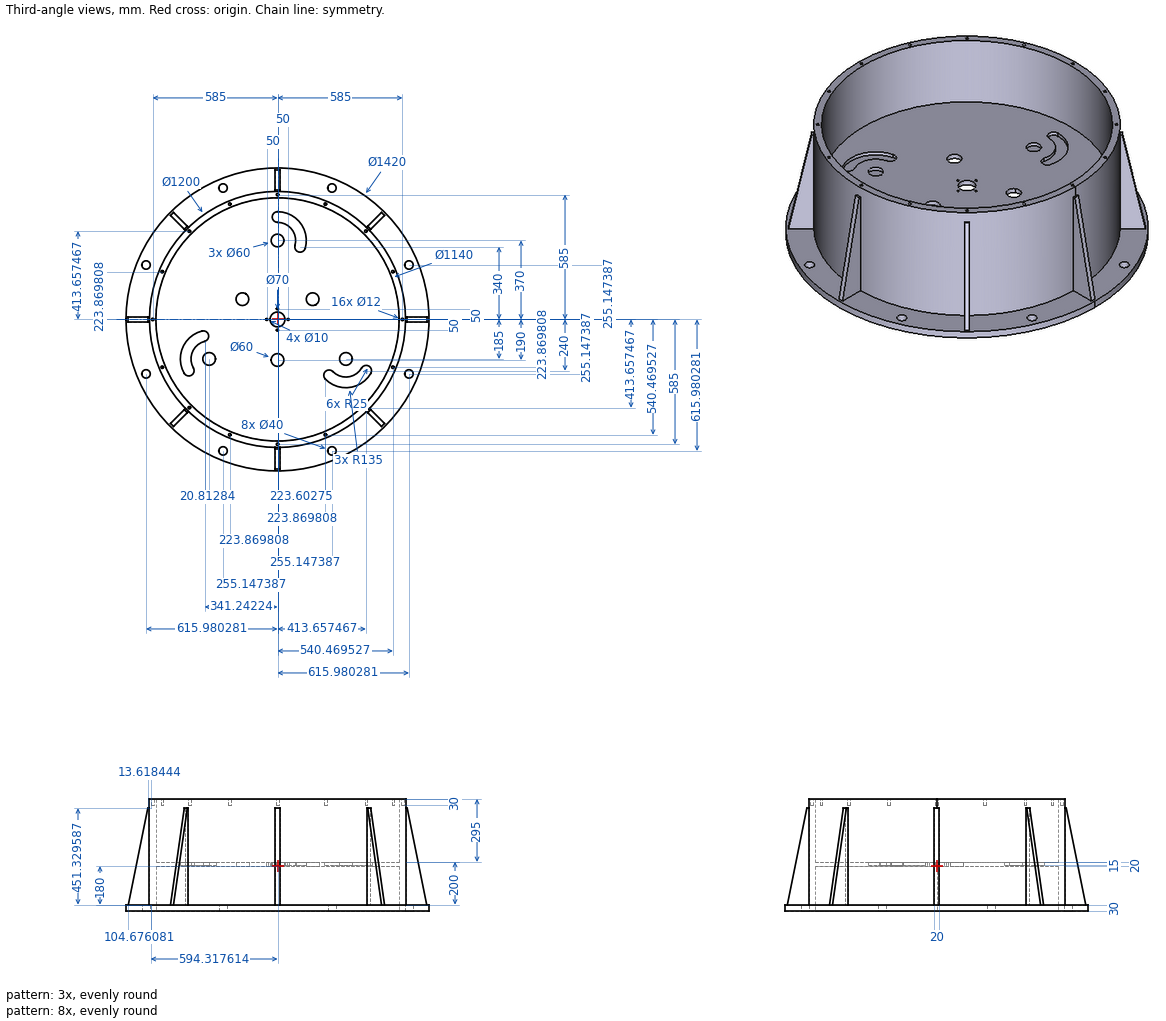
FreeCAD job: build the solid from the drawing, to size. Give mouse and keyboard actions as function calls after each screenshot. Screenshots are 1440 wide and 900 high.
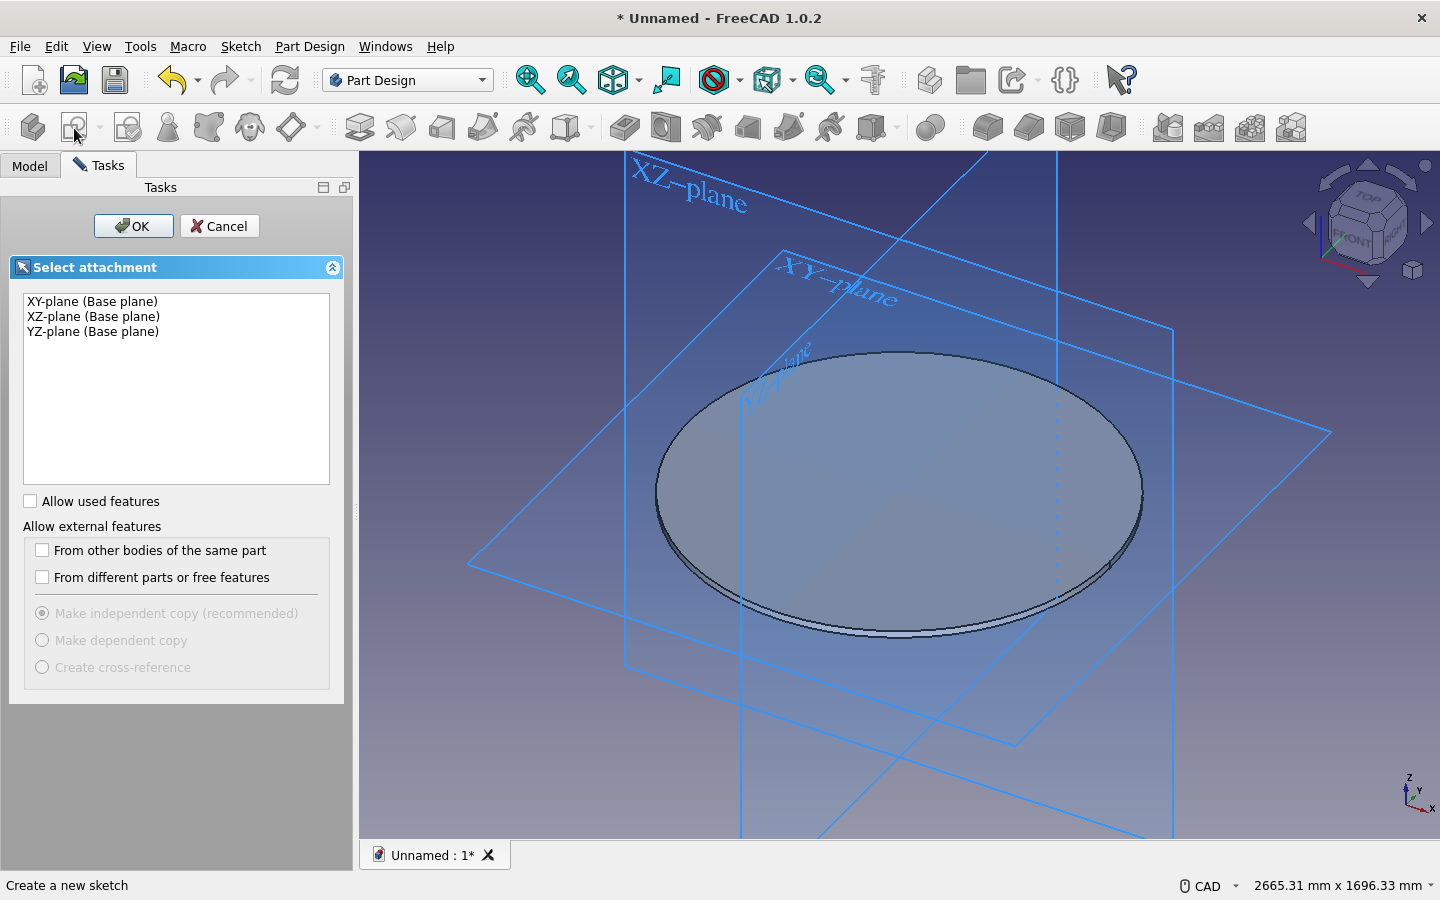
click(84, 302)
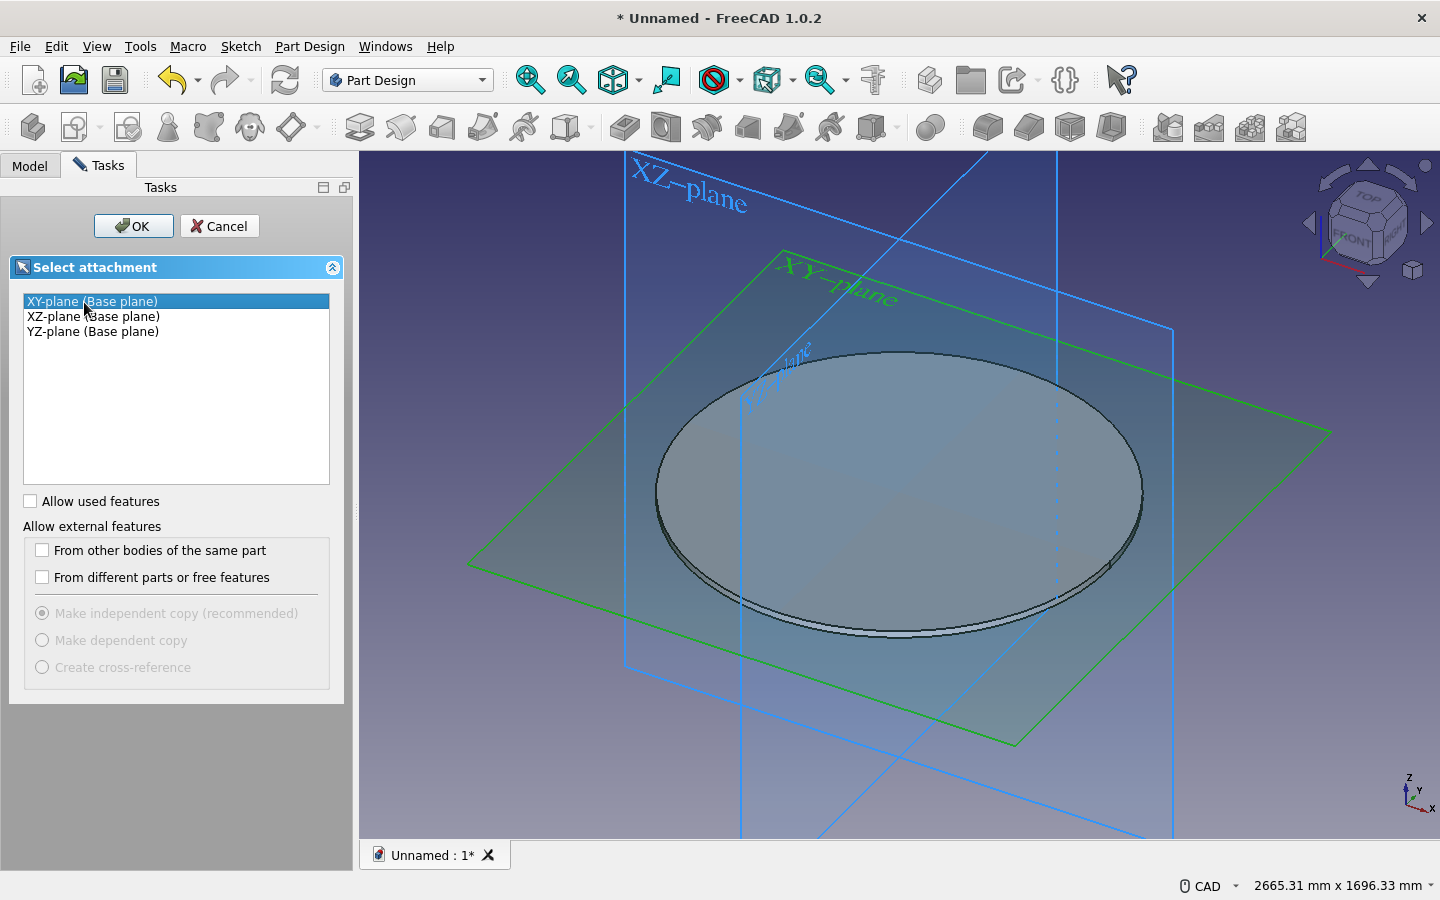
click(134, 226)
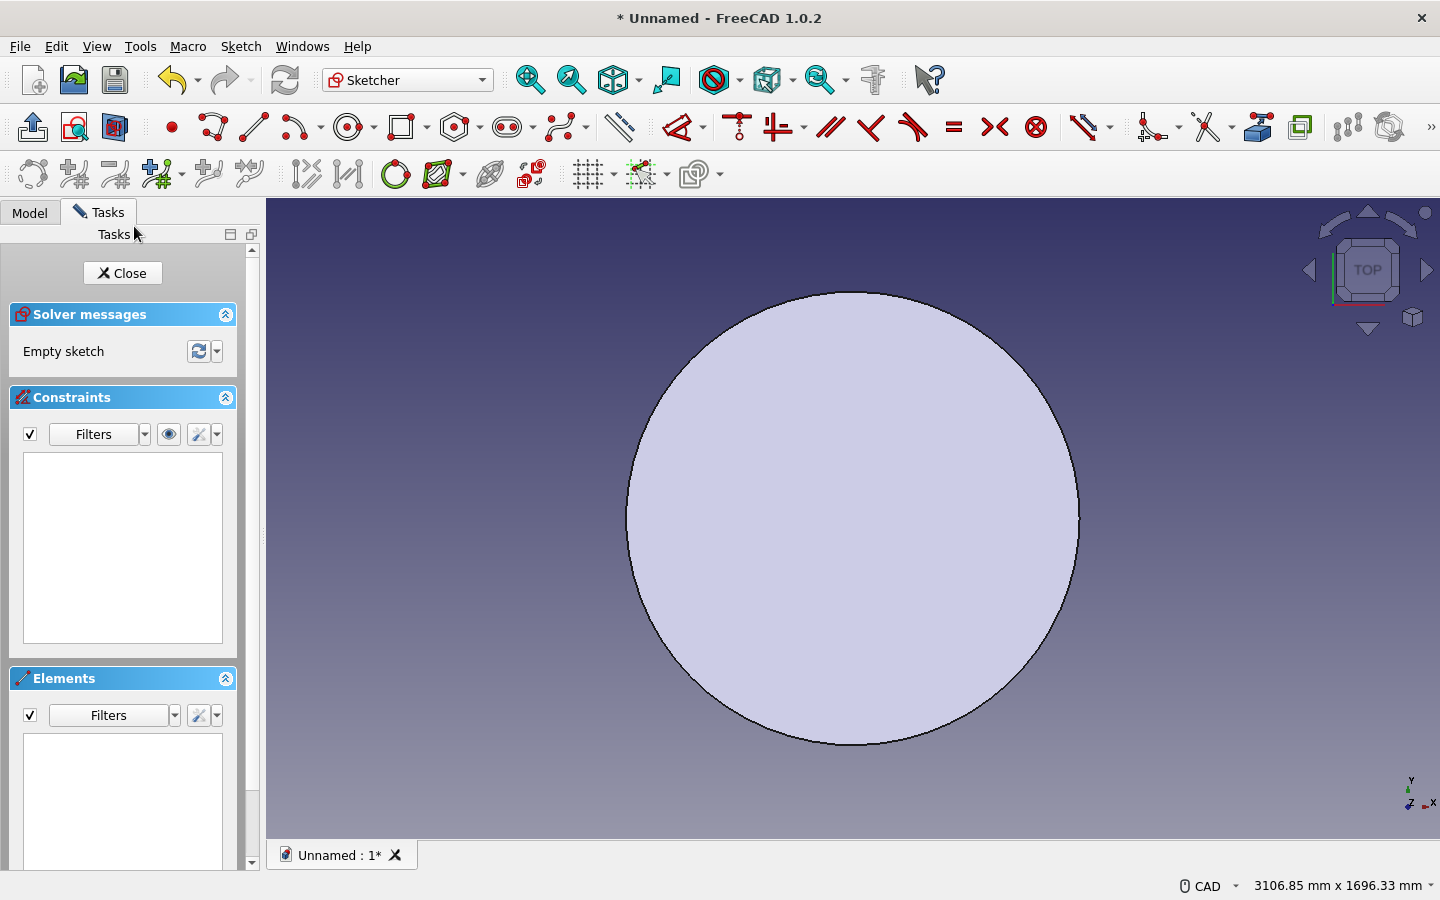
key(q)
key(s)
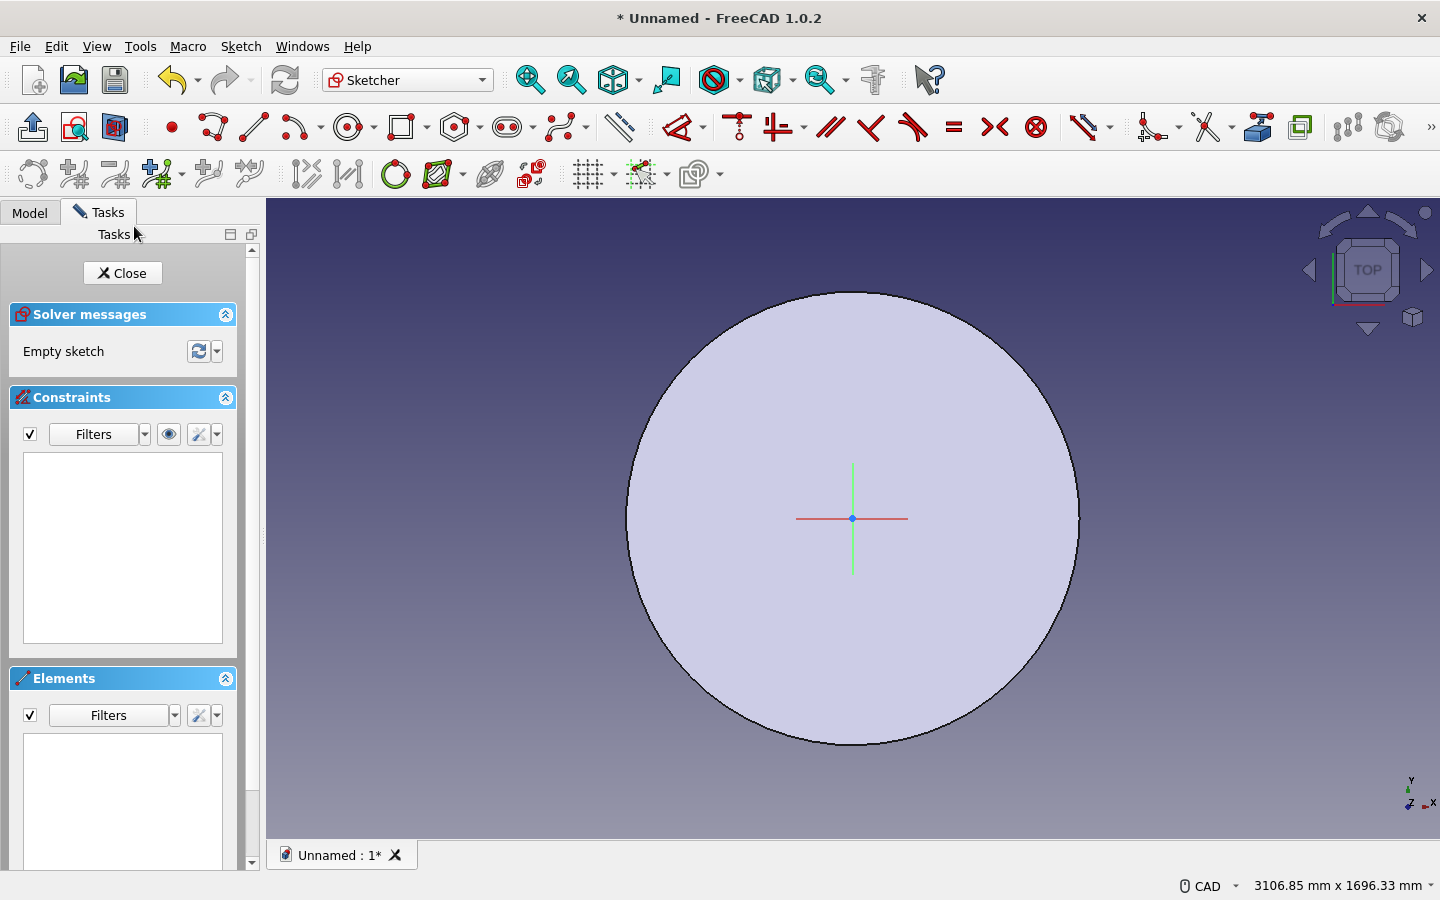
scroll(861, 518, up, 11)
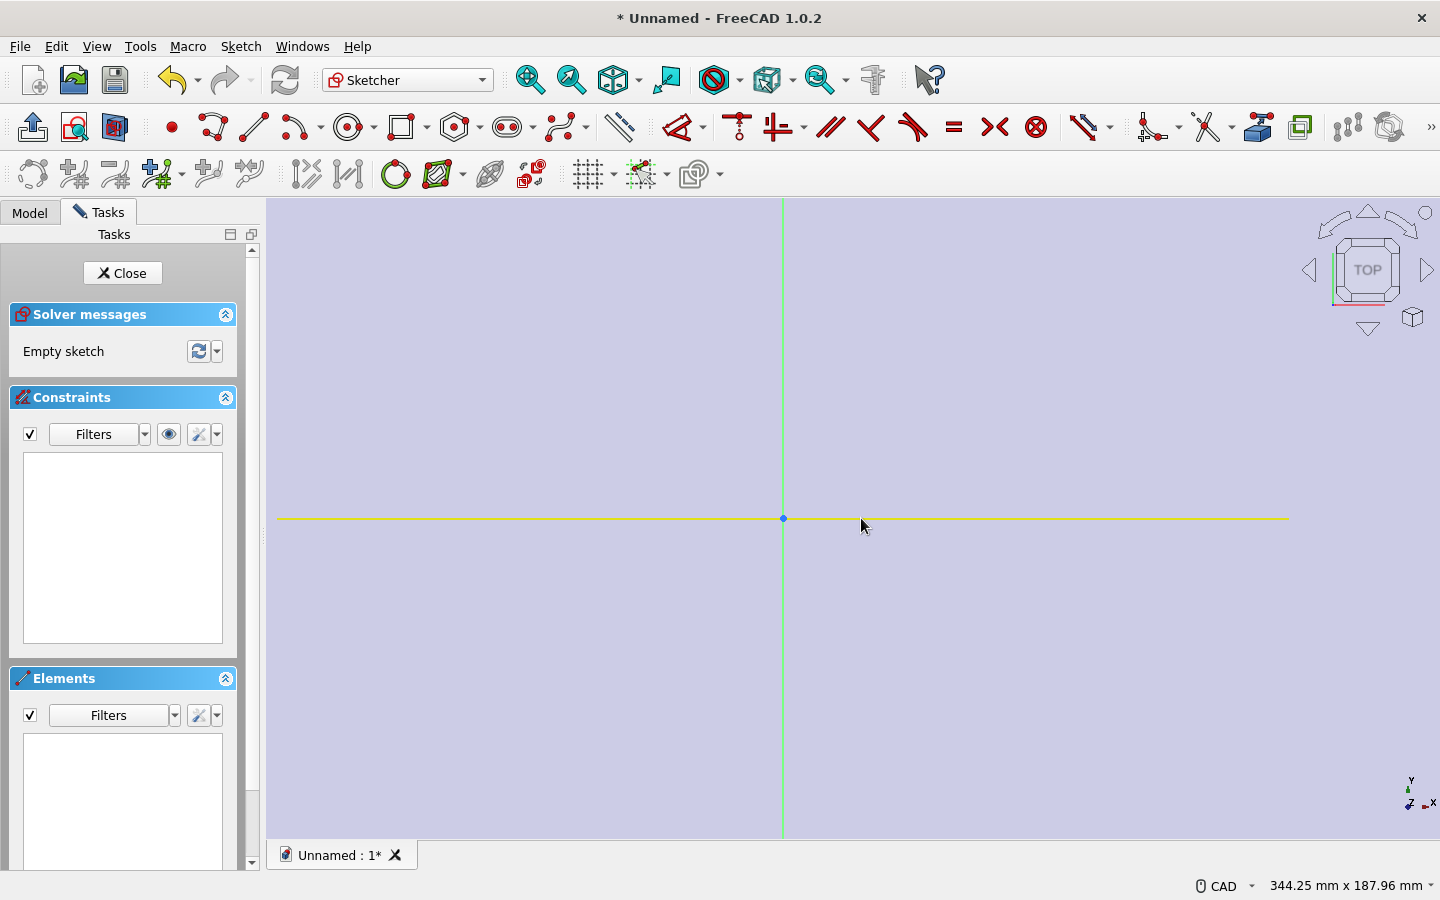
key(g)
key(c)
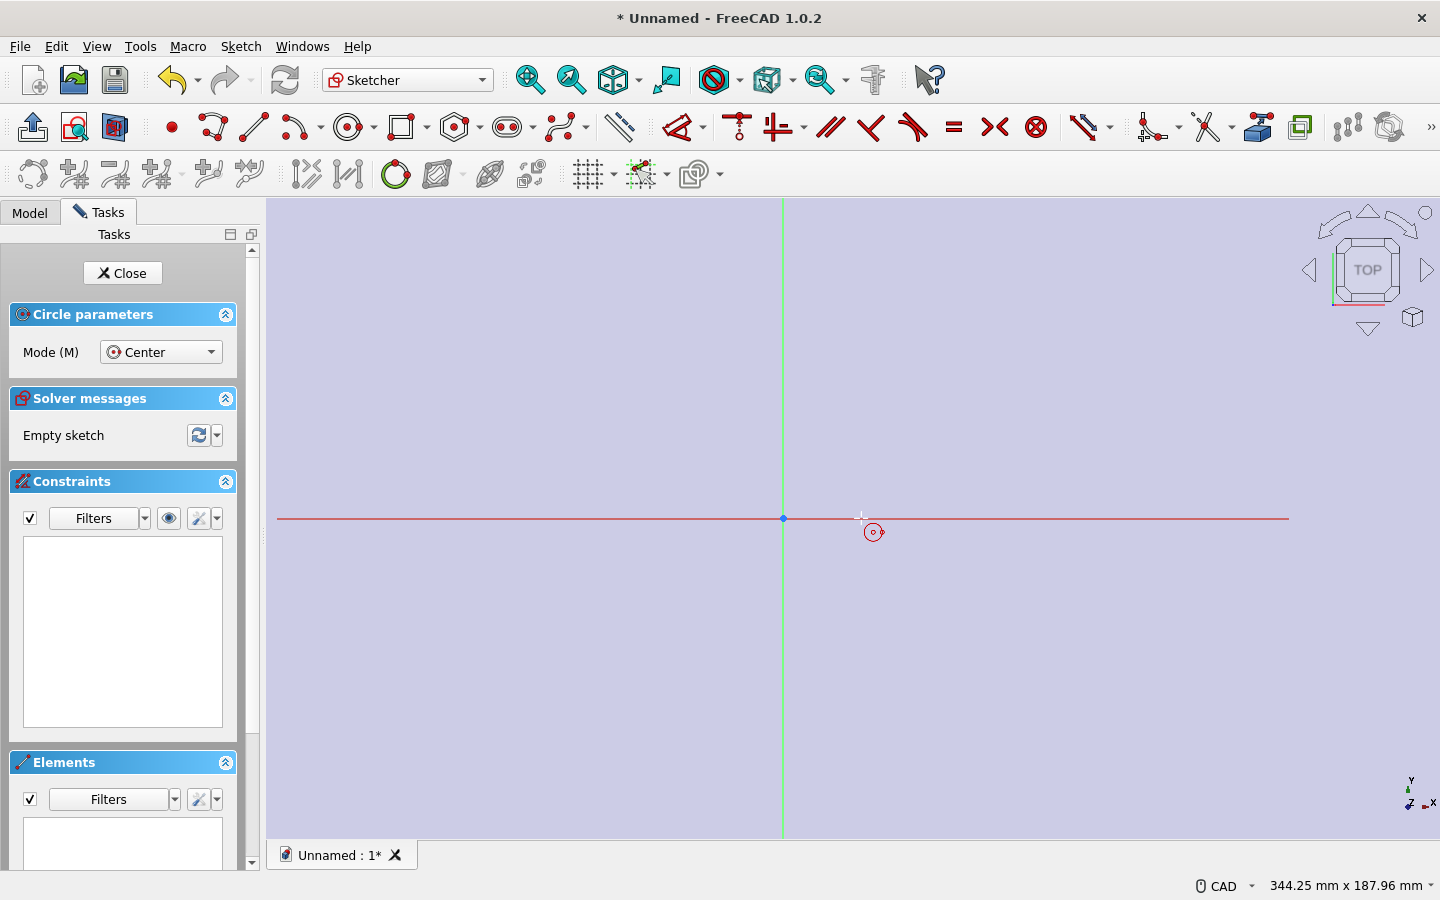
click(783, 518)
move(868, 434)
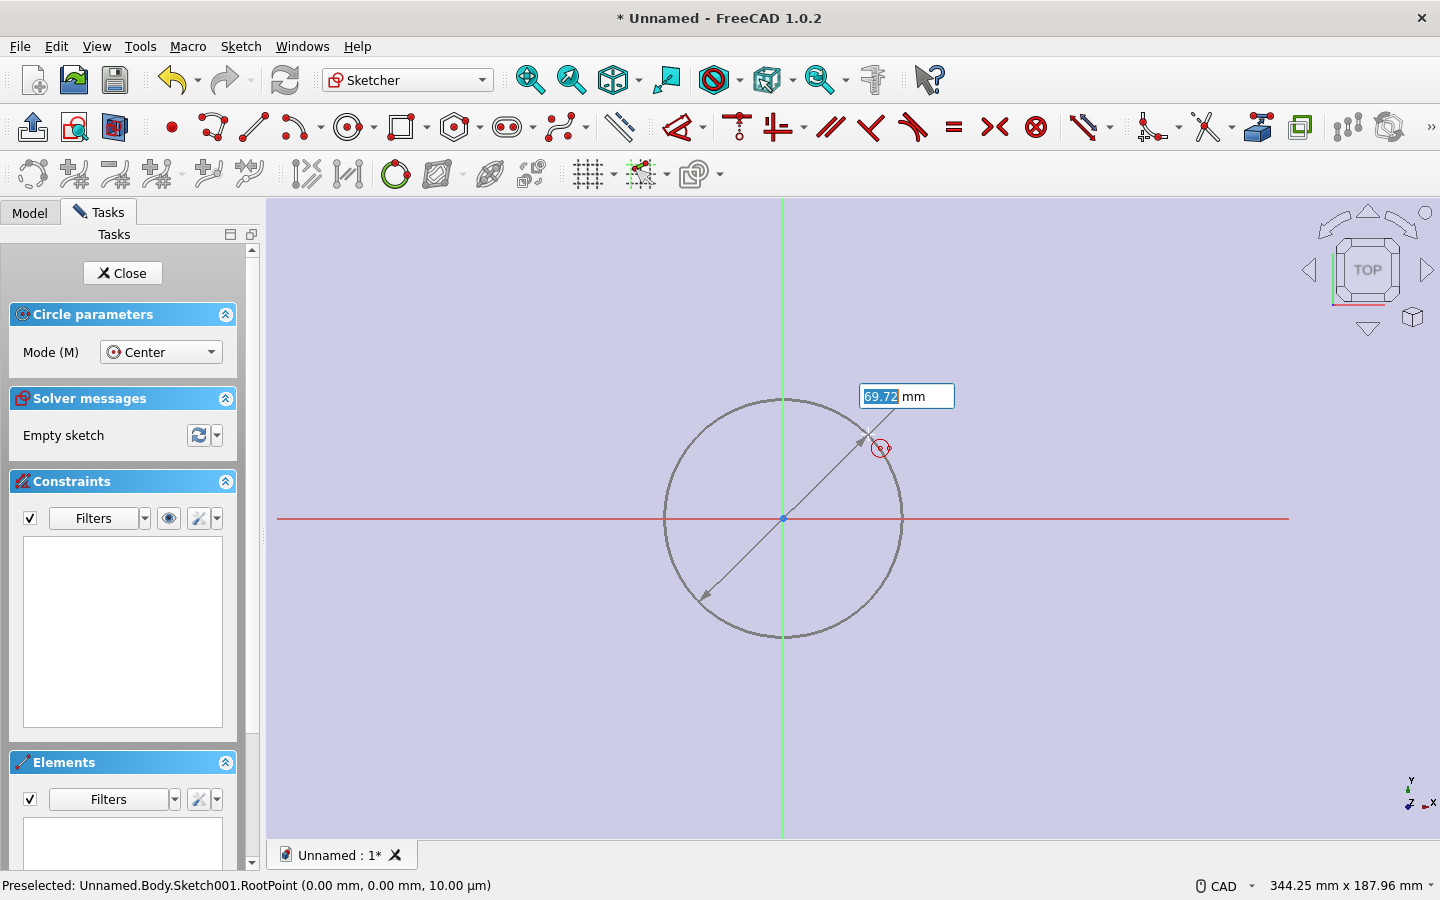
text(70)
key(Return)